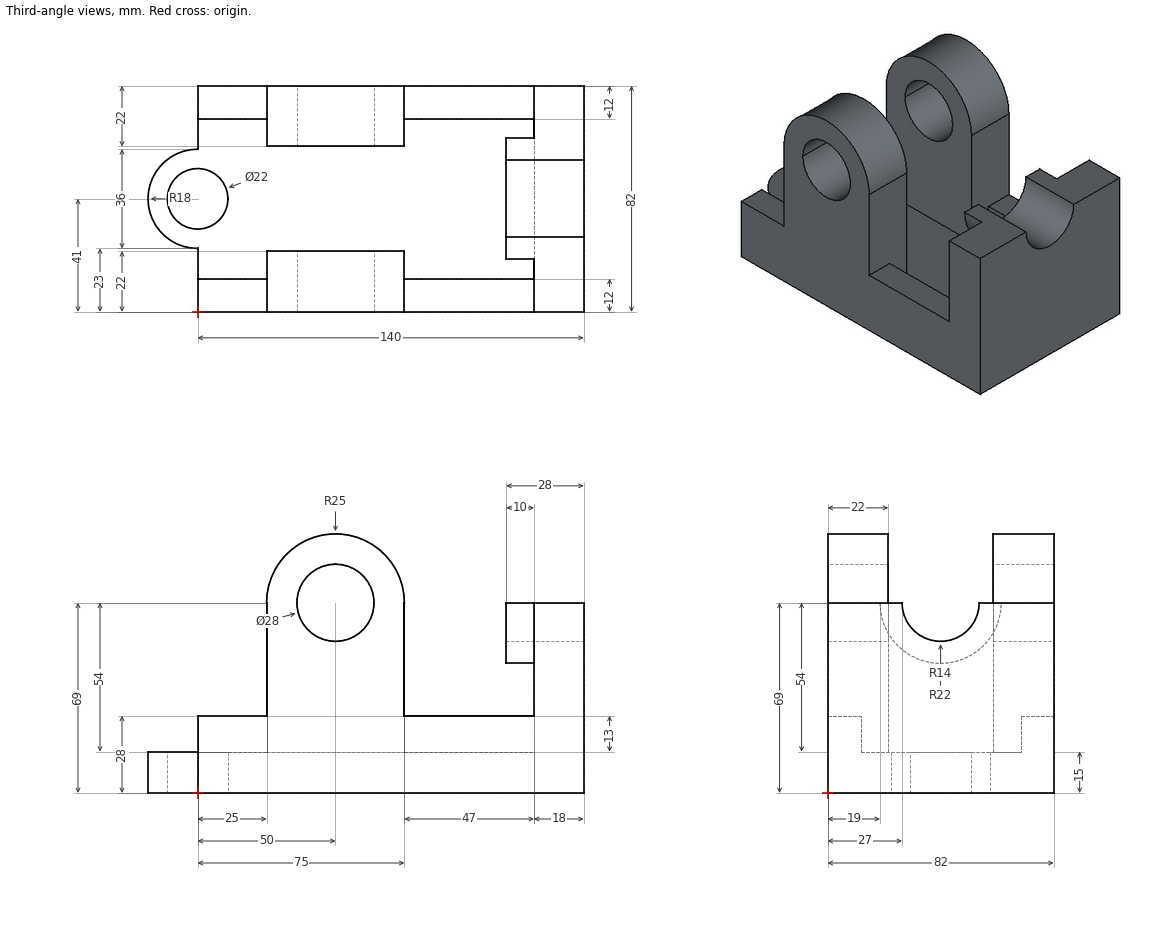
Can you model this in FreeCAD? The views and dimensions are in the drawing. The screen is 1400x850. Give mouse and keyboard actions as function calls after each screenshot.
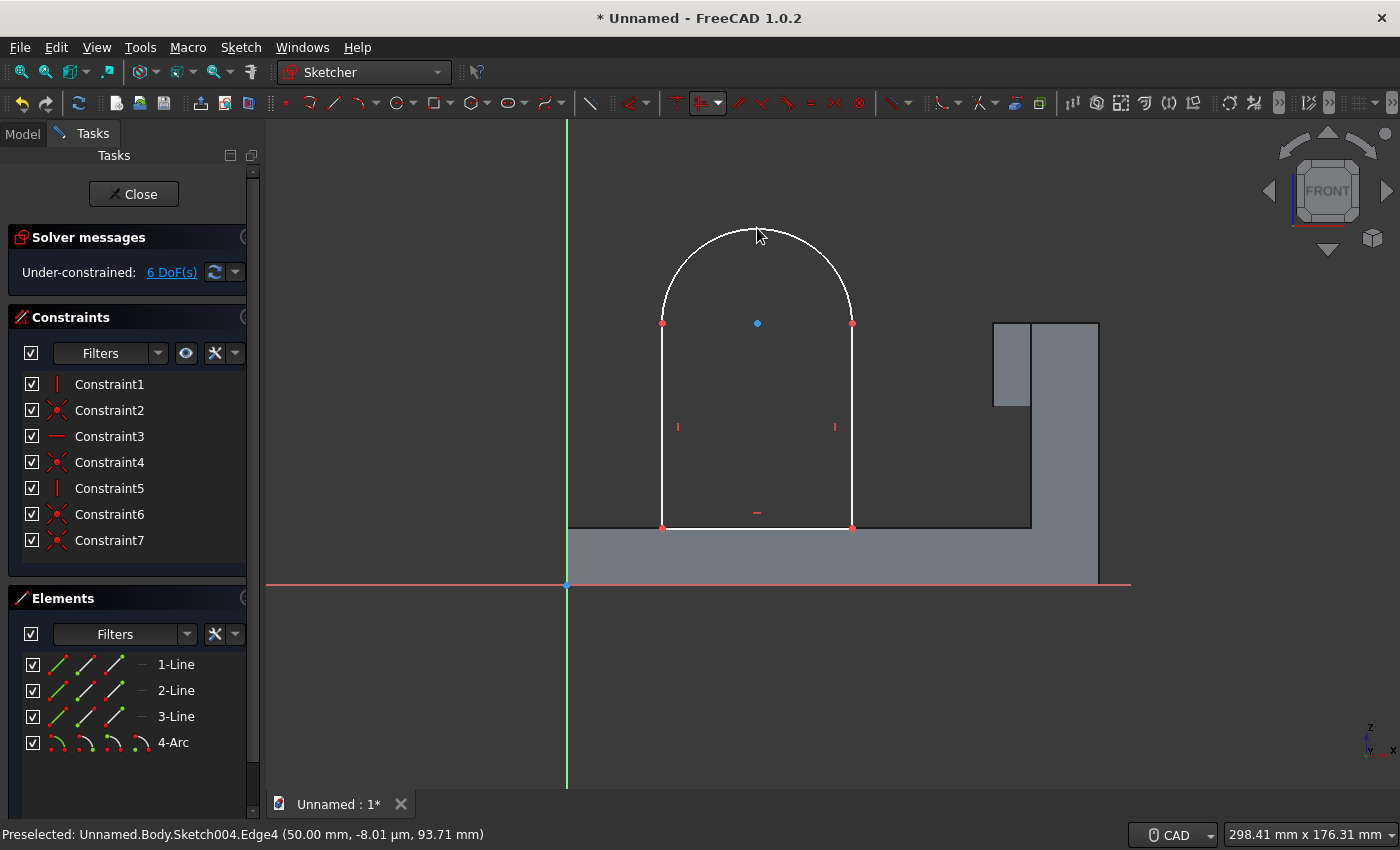
click(662, 385)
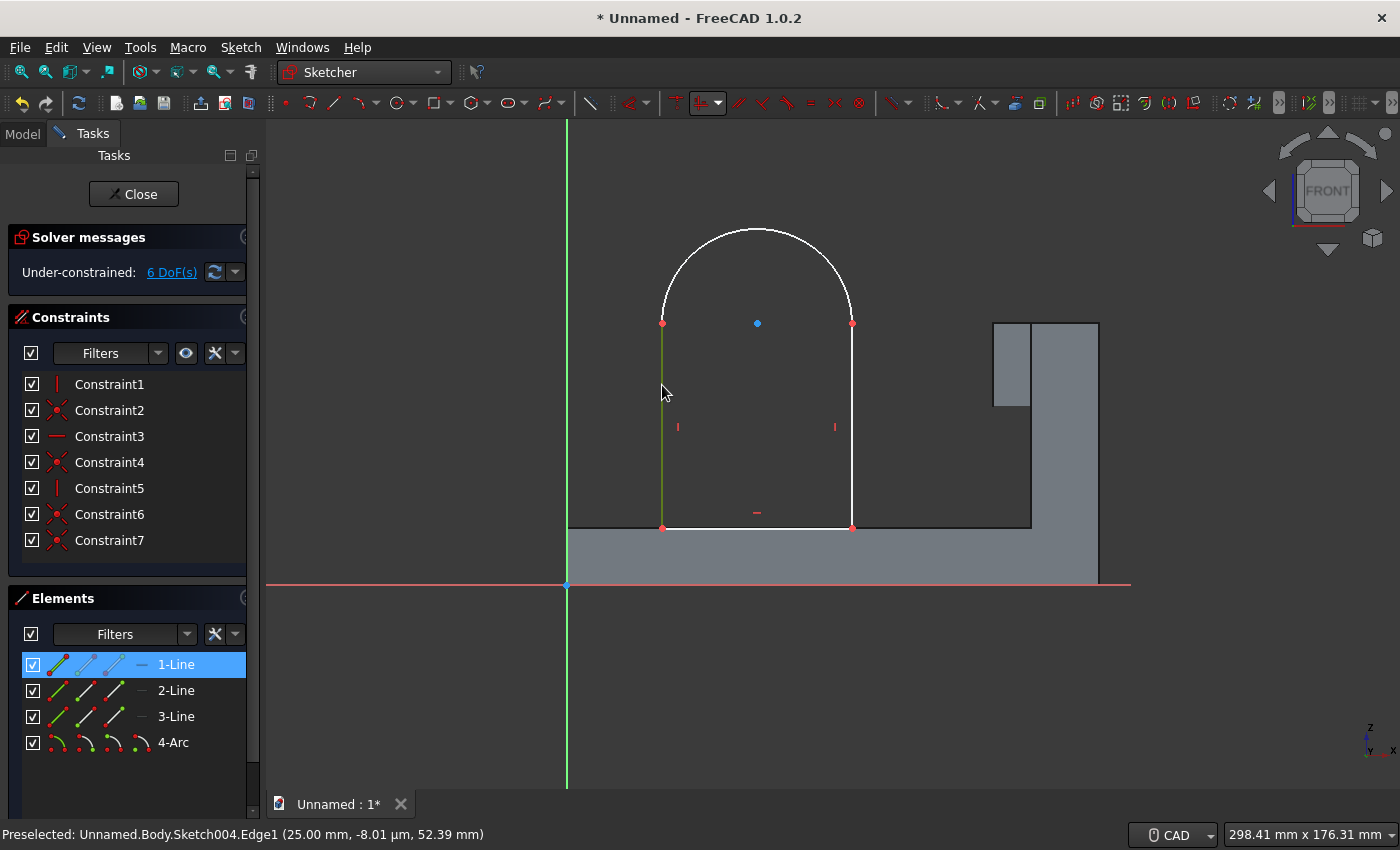
click(813, 247)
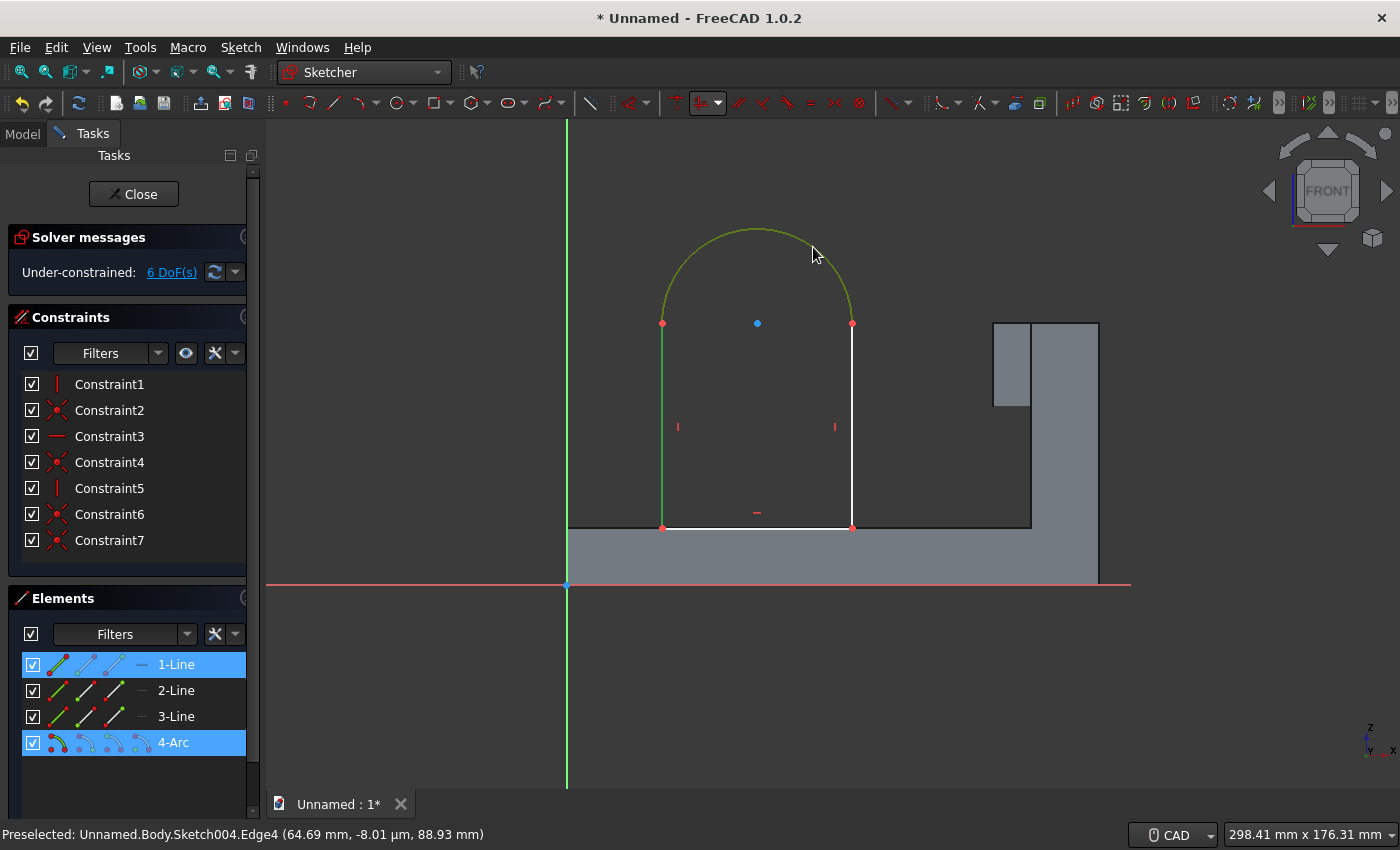
click(788, 104)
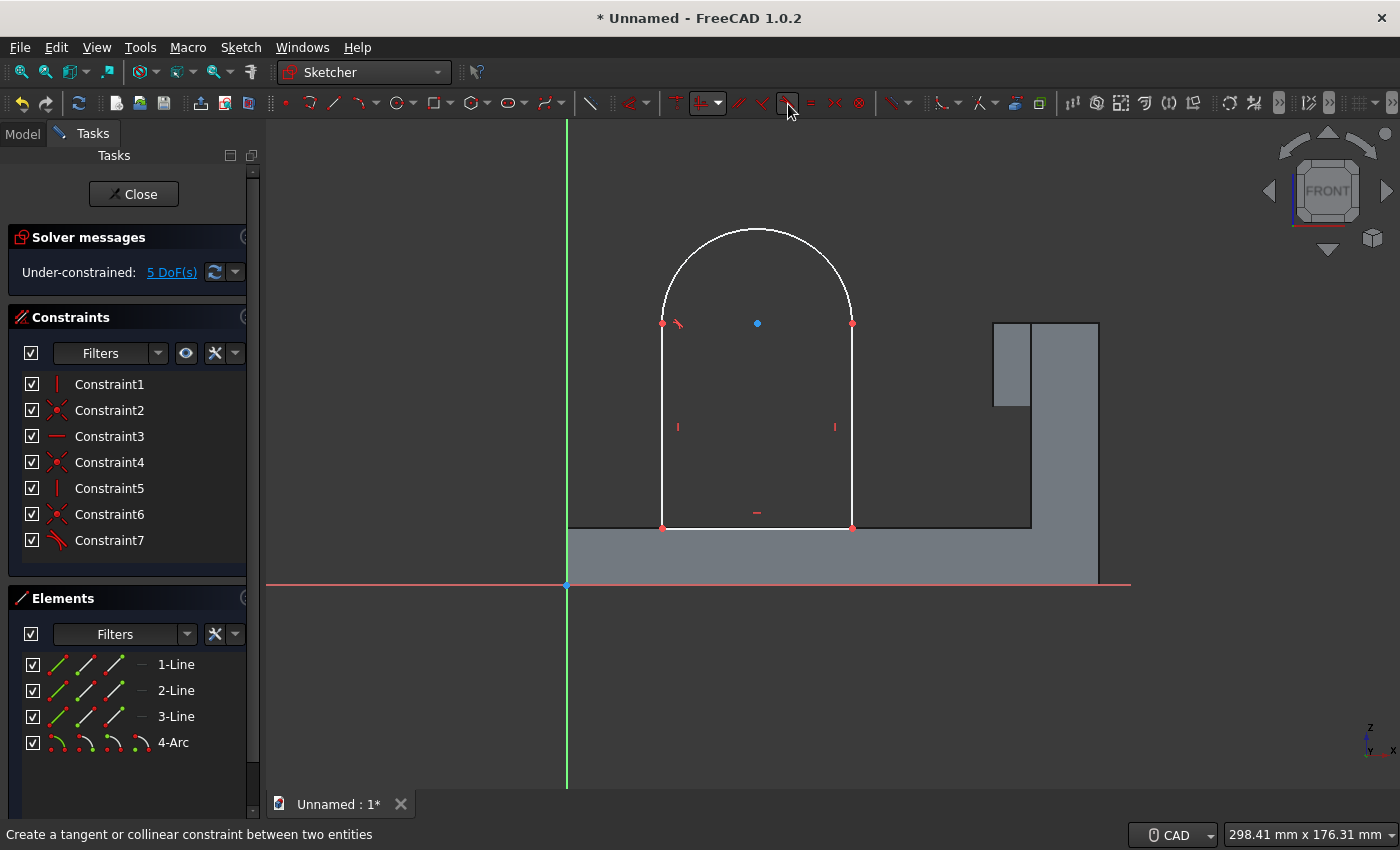
click(852, 467)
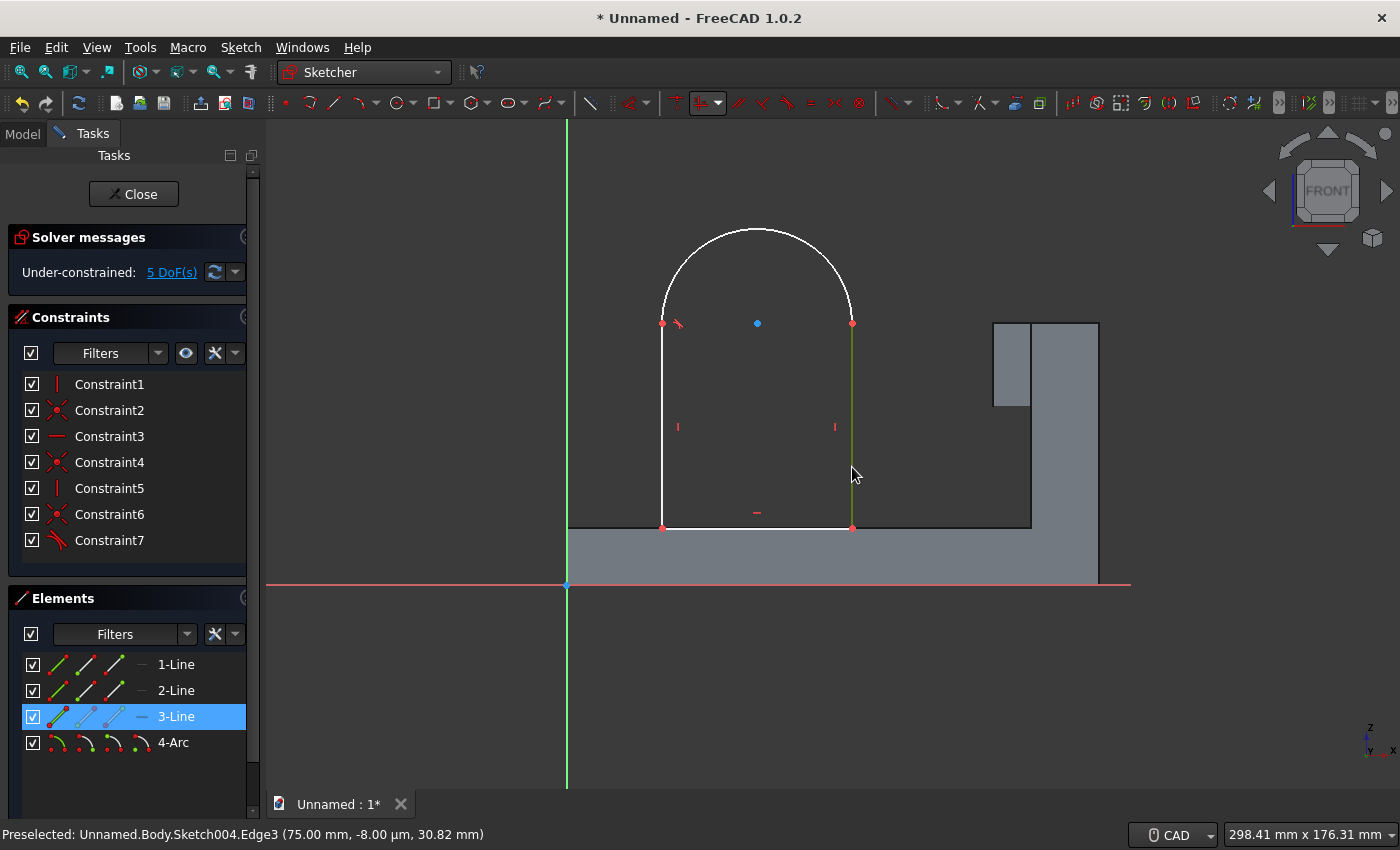
click(813, 247)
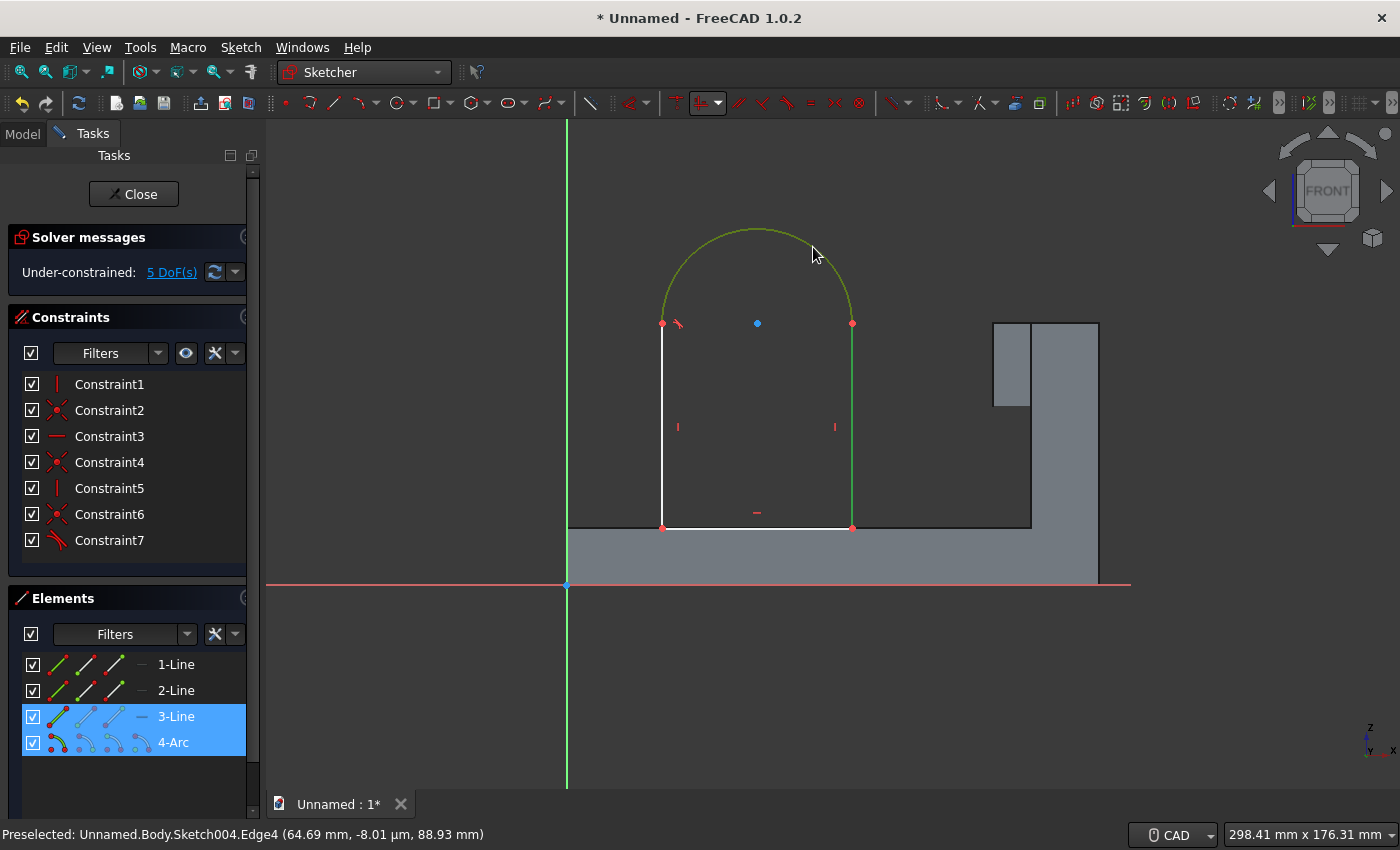
click(788, 104)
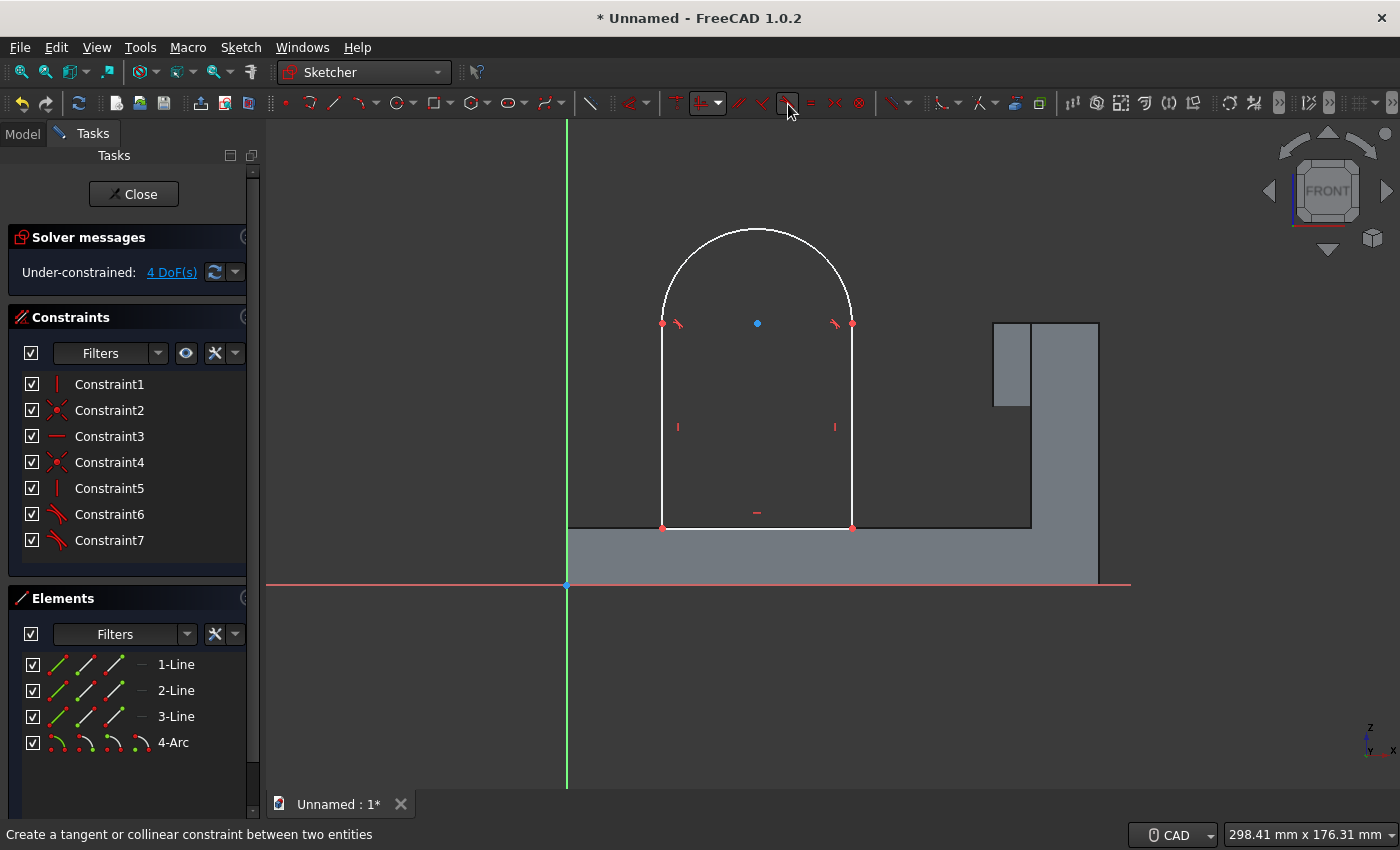
click(630, 104)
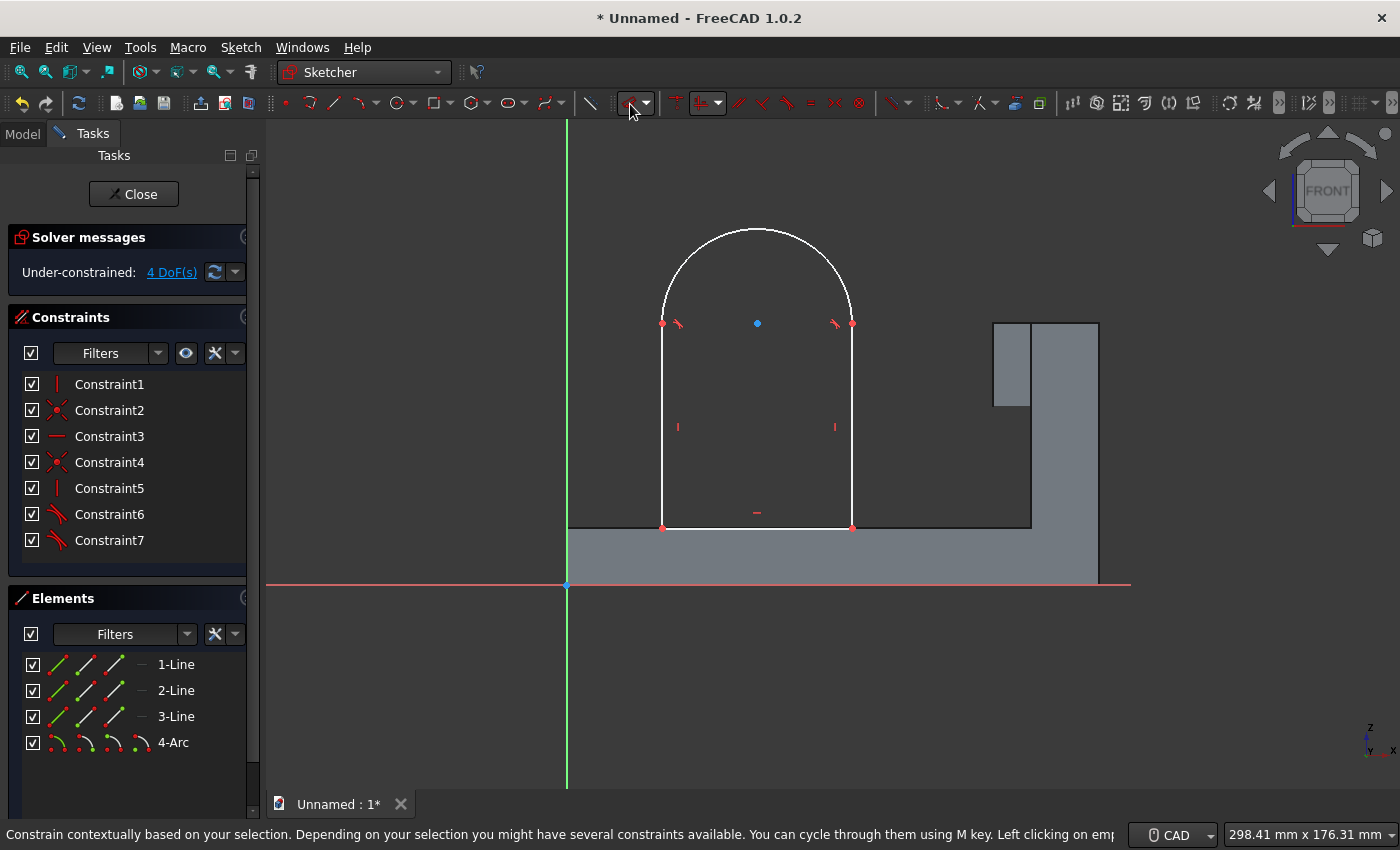
click(813, 247)
click(832, 221)